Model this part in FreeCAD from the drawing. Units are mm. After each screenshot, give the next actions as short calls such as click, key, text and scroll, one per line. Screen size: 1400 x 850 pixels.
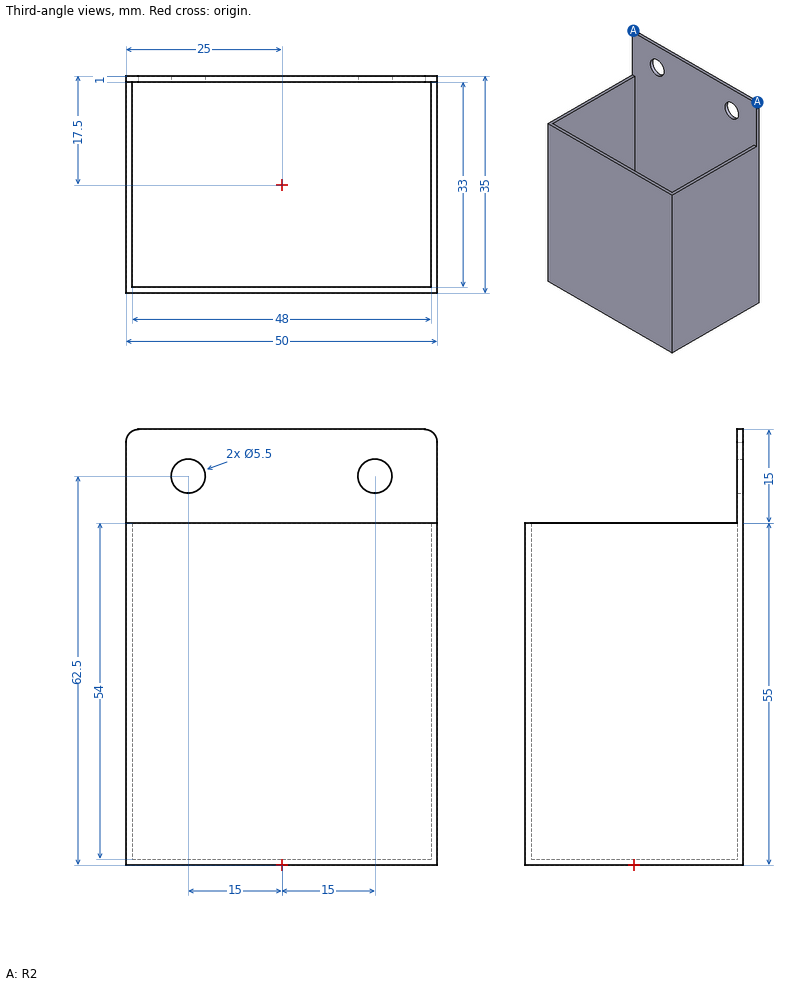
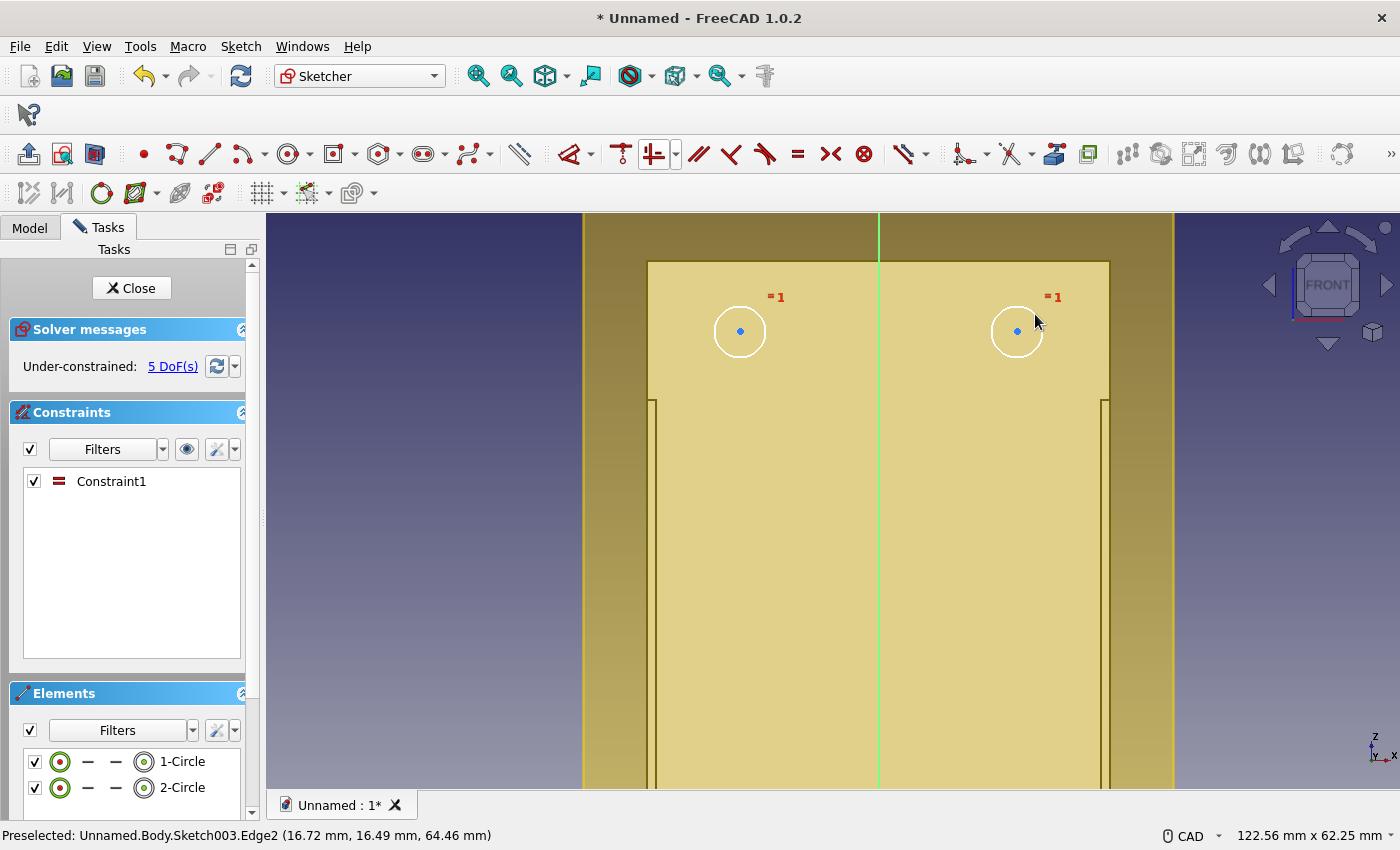
click(740, 332)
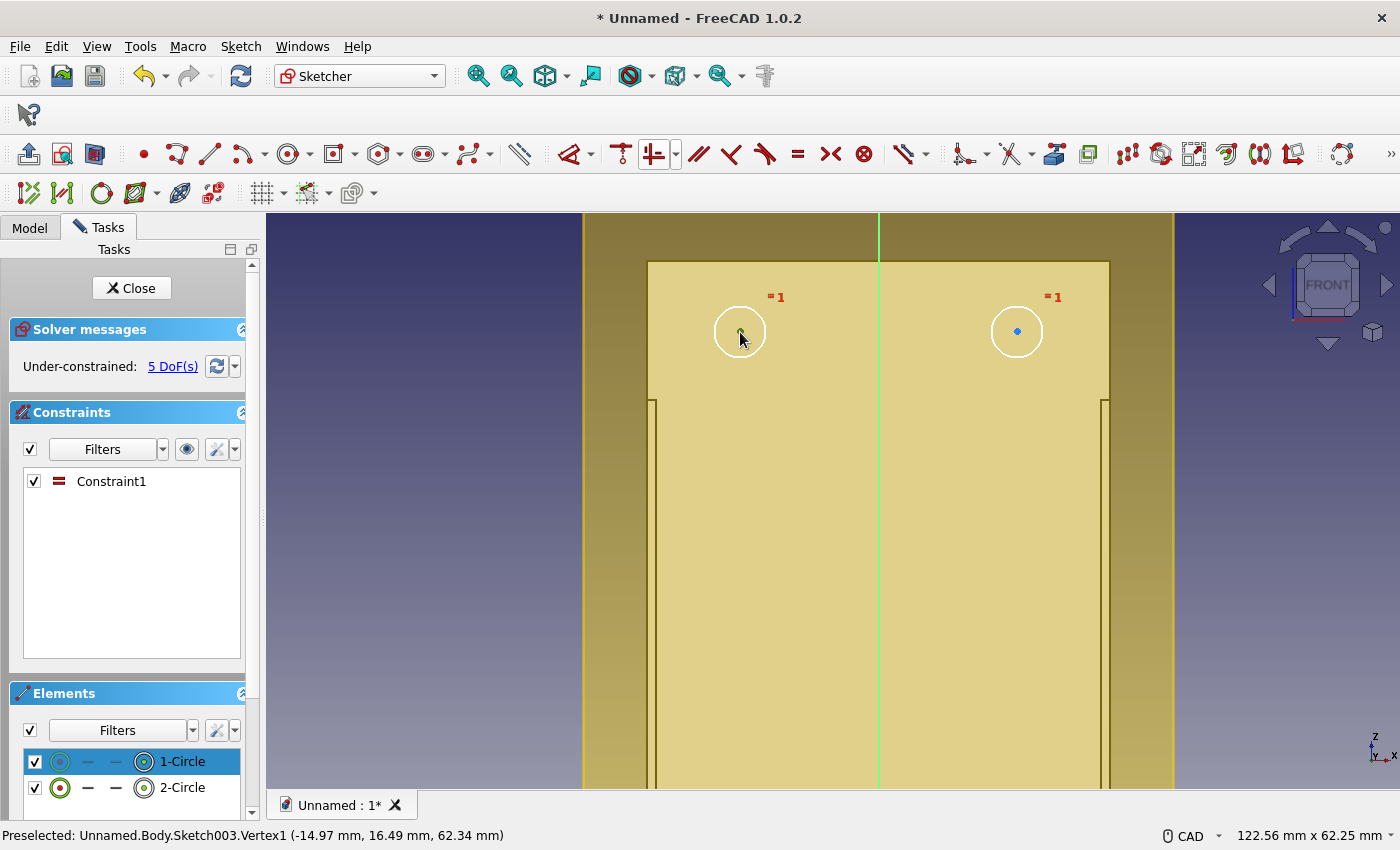
click(1017, 332)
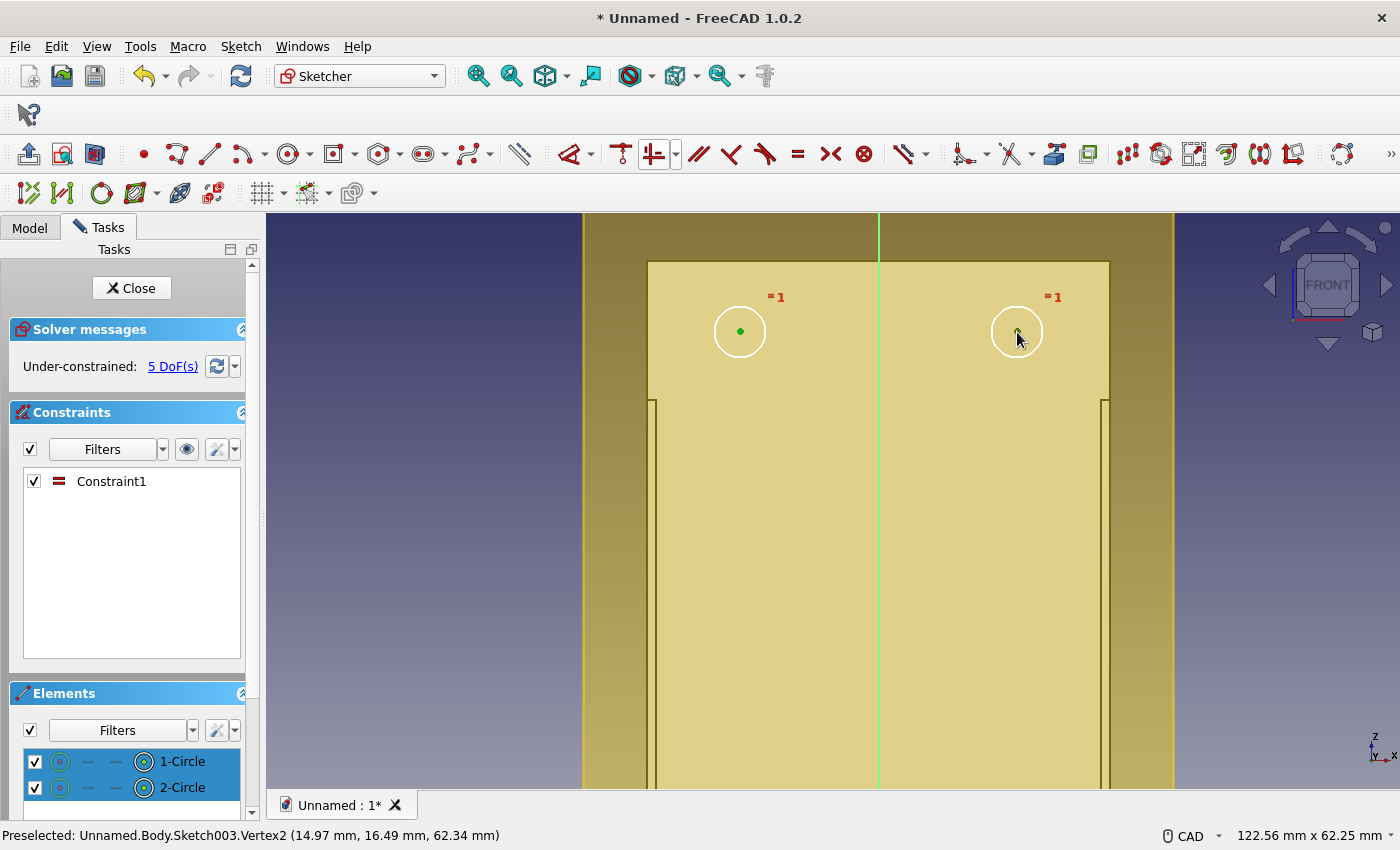
key(h)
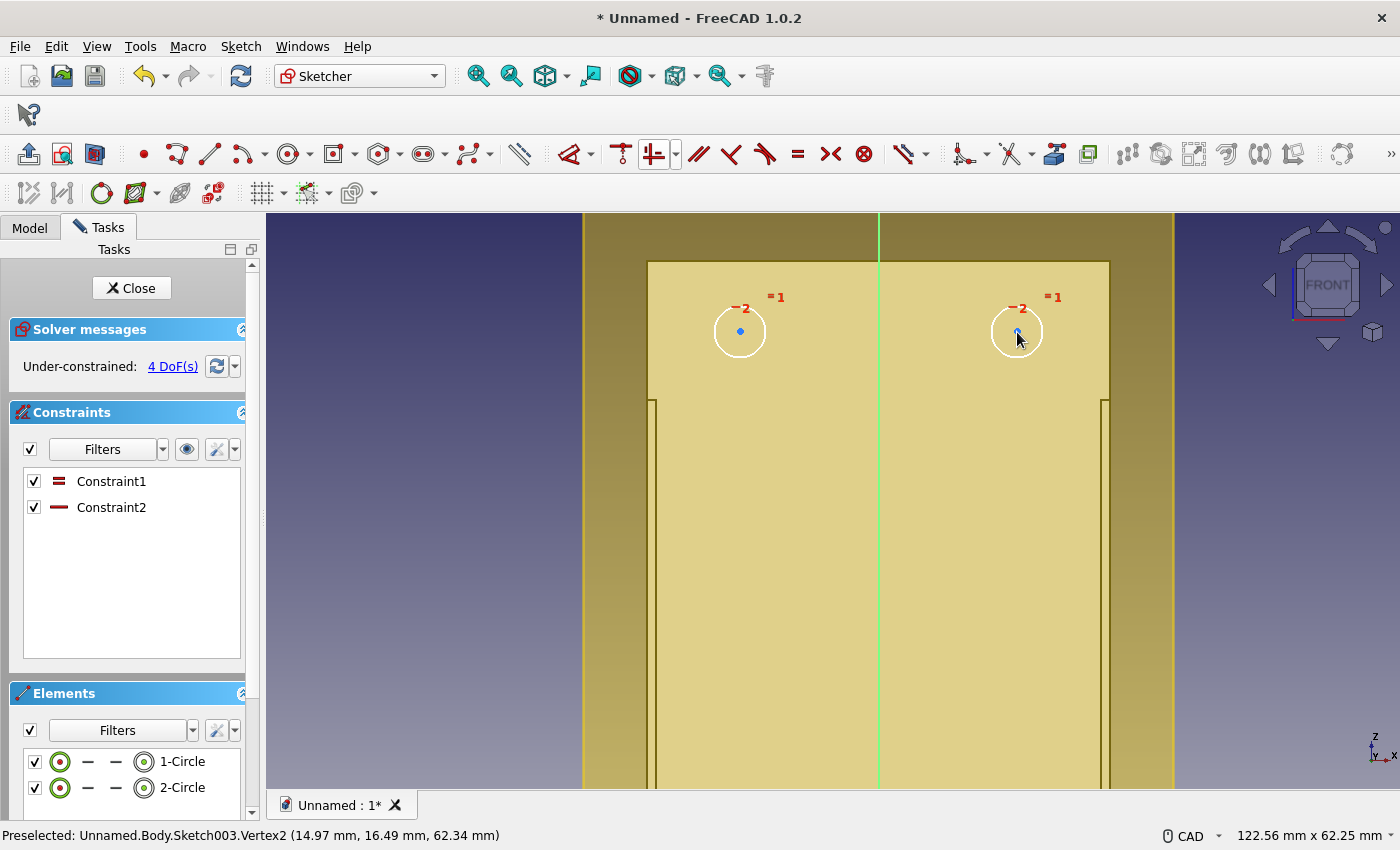
key(d)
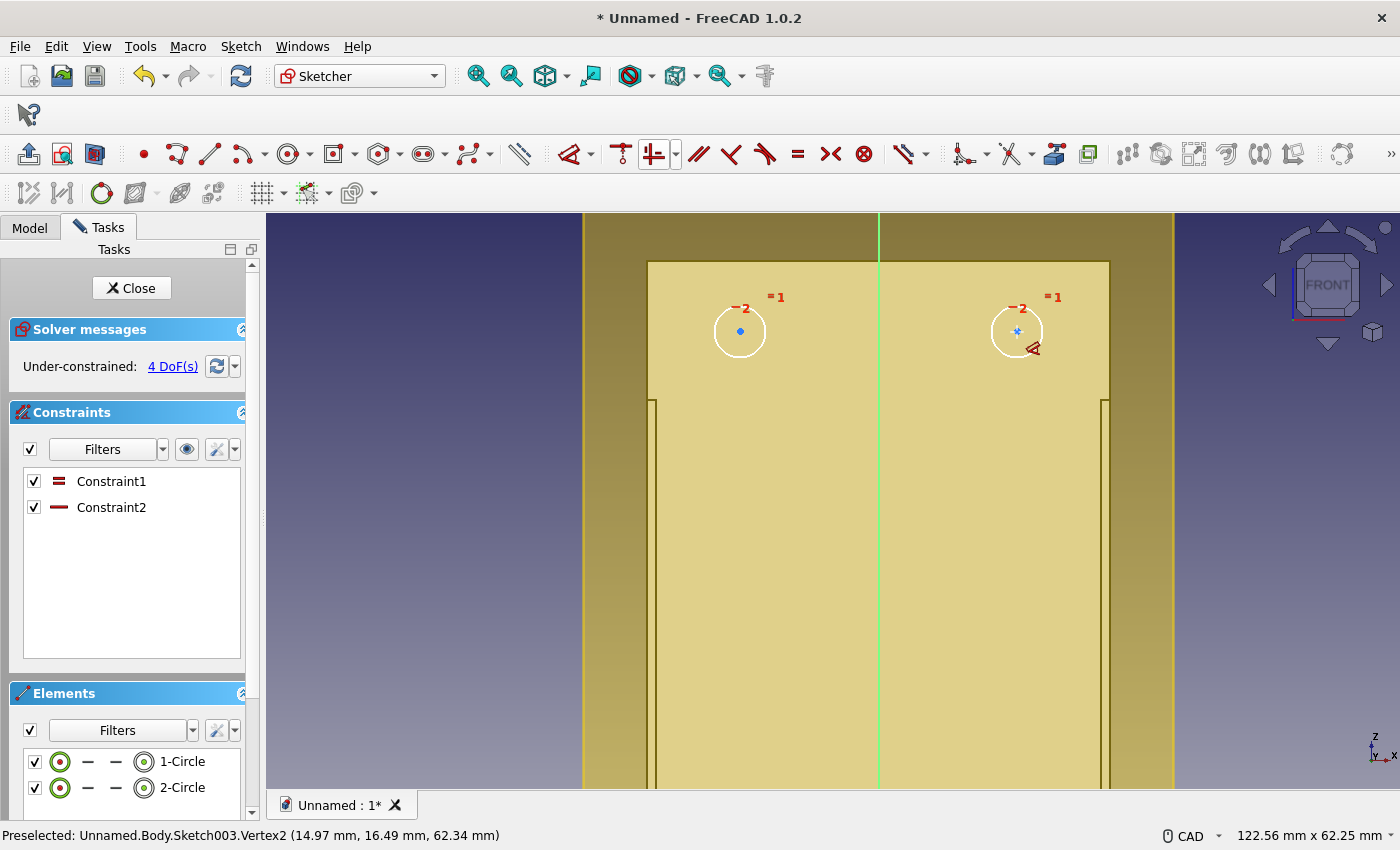
click(758, 314)
click(781, 291)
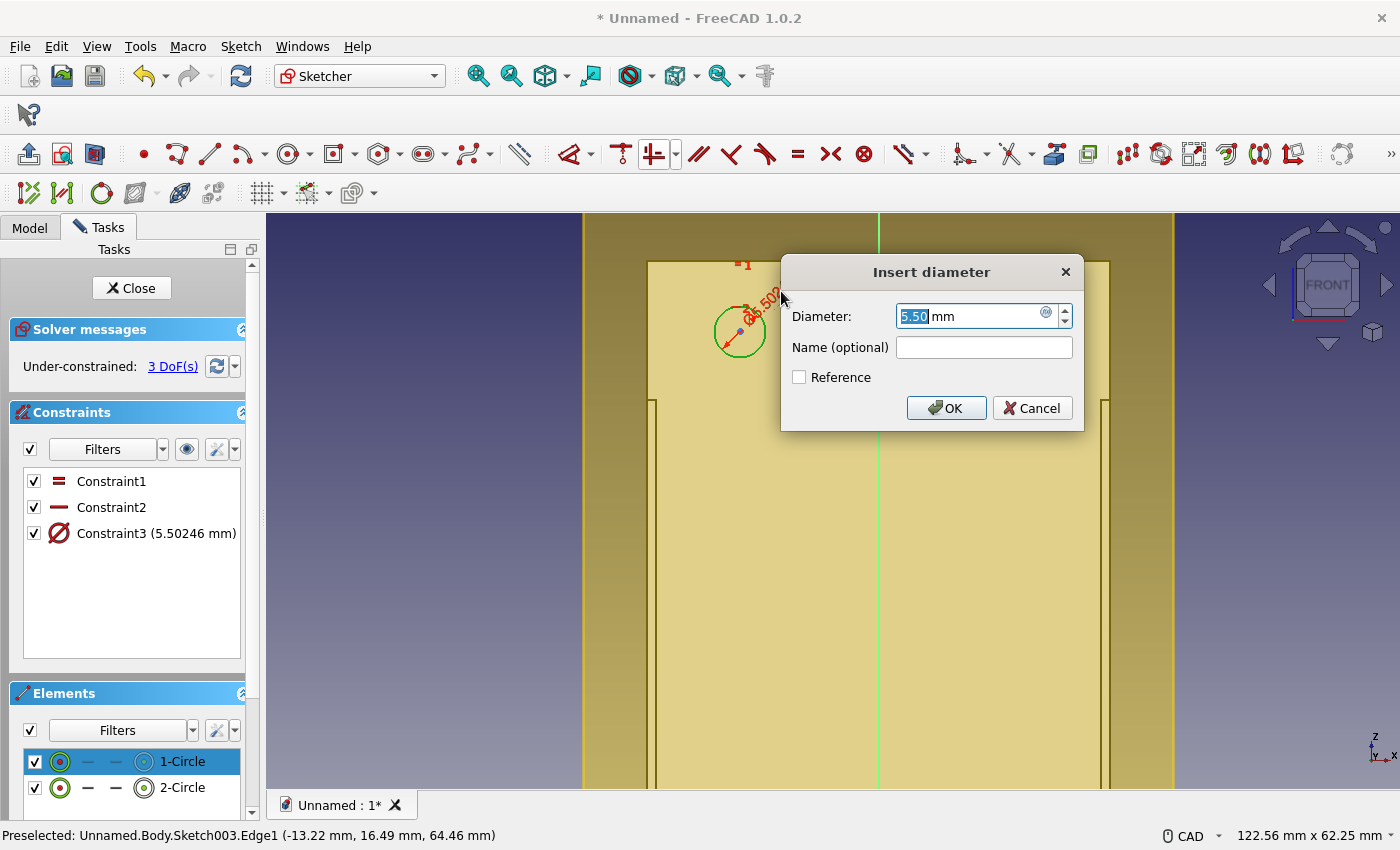
text(5.5)
key(Return)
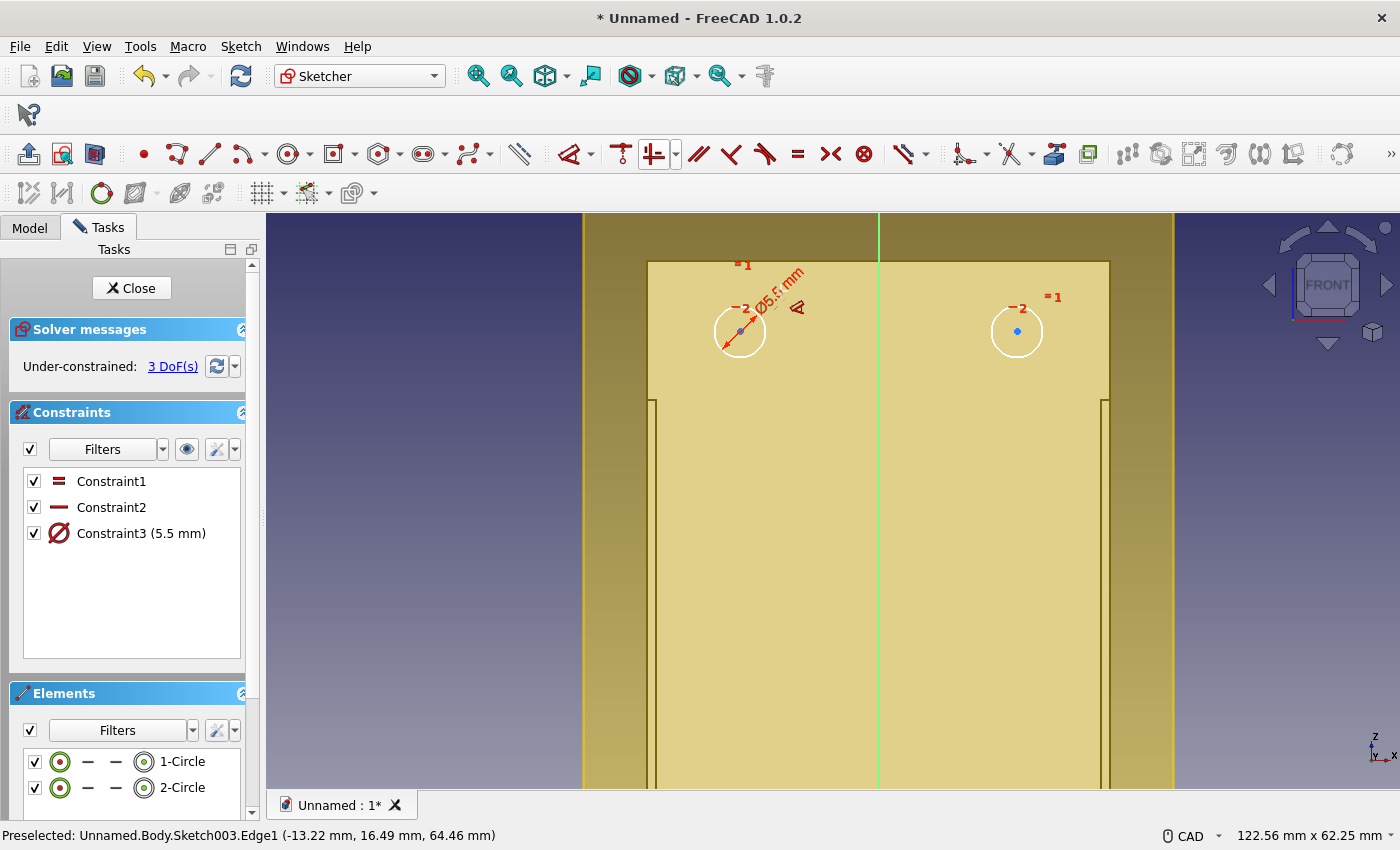
click(740, 332)
click(858, 298)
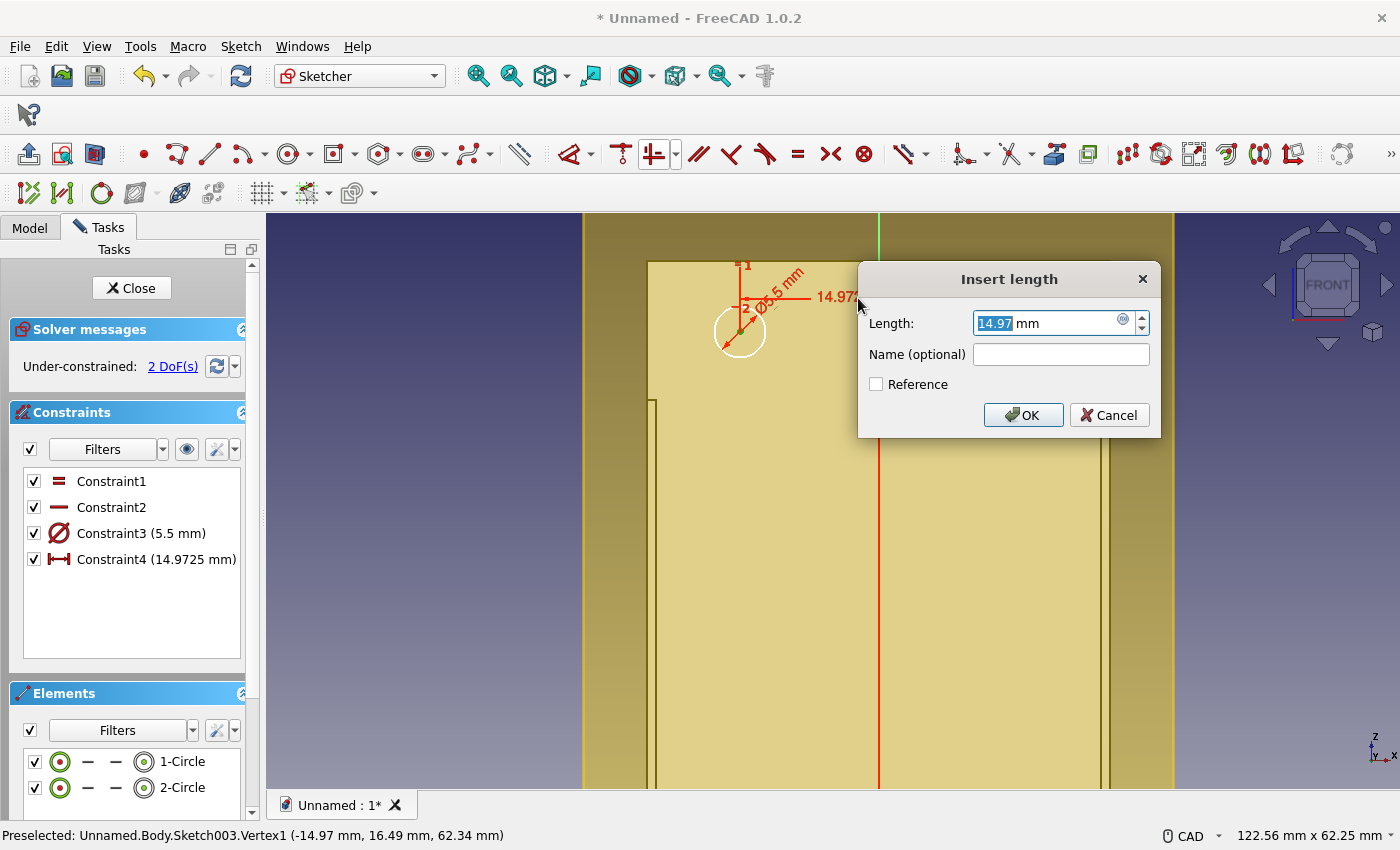
text(15)
key(Return)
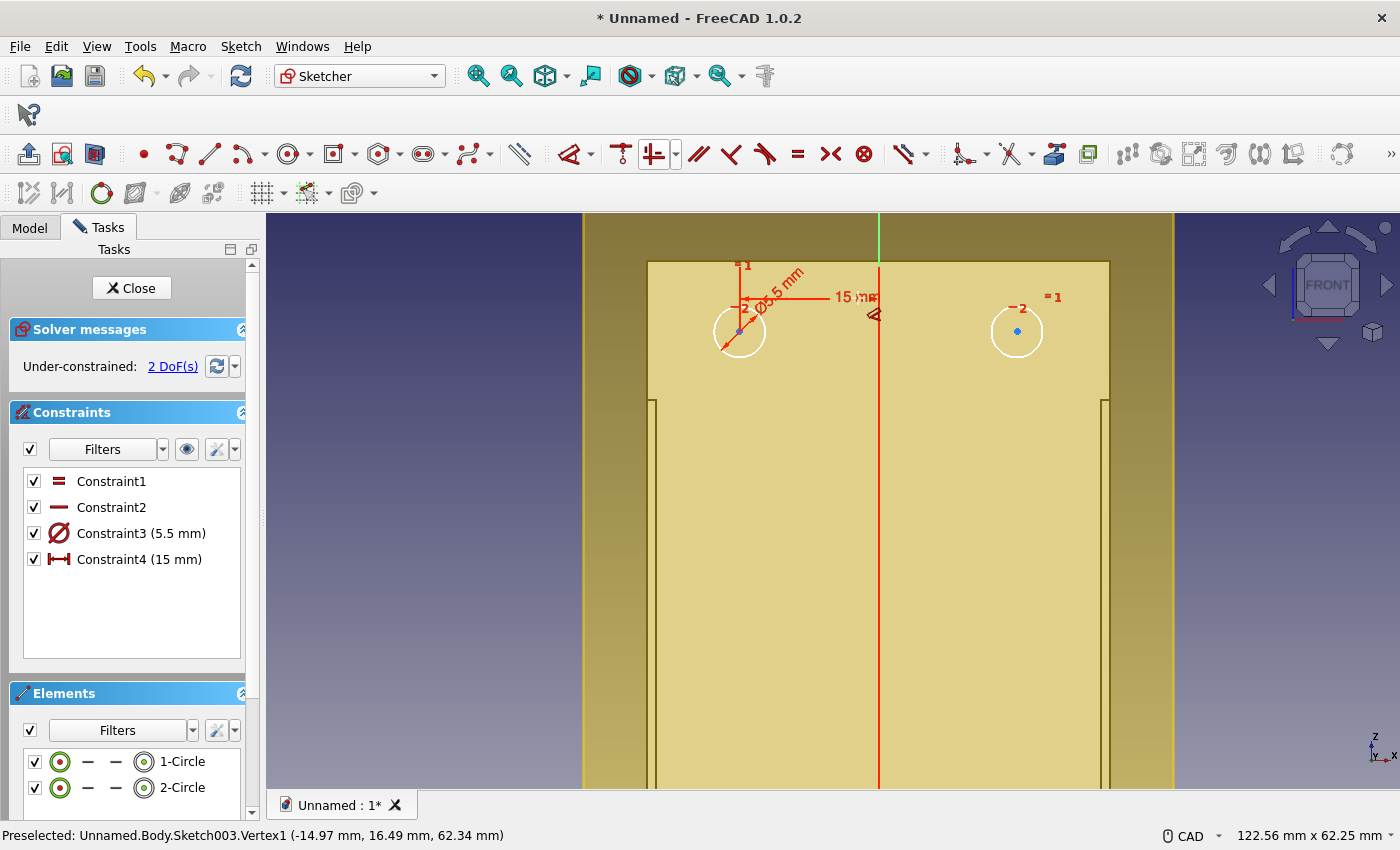
click(1017, 332)
click(948, 298)